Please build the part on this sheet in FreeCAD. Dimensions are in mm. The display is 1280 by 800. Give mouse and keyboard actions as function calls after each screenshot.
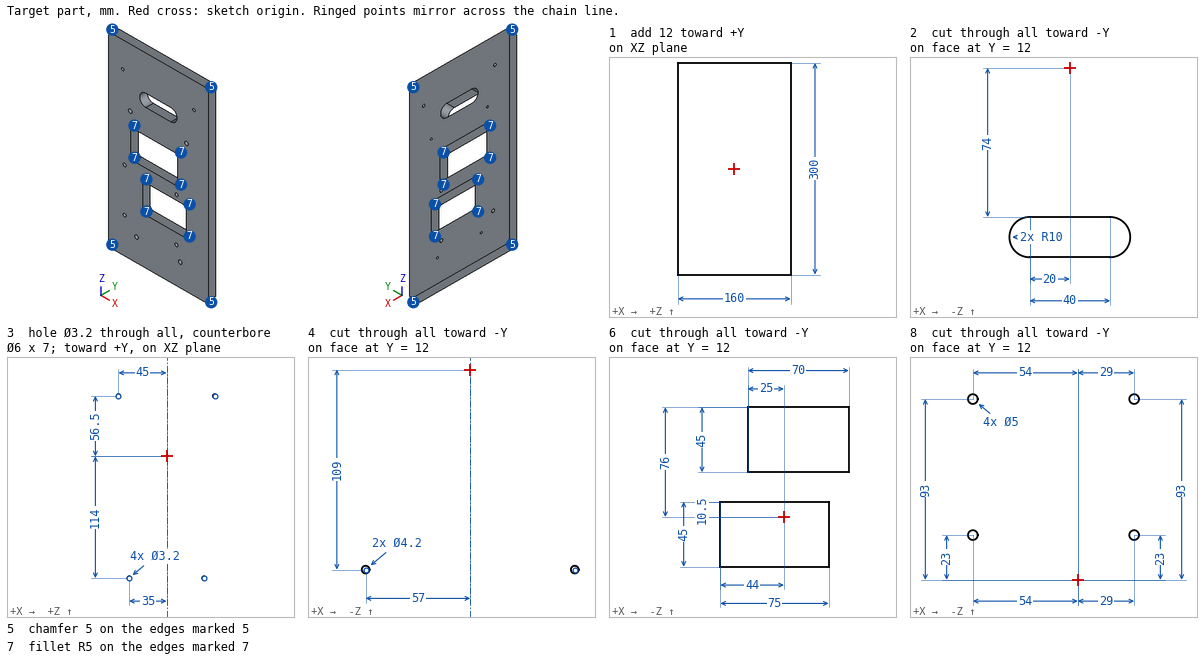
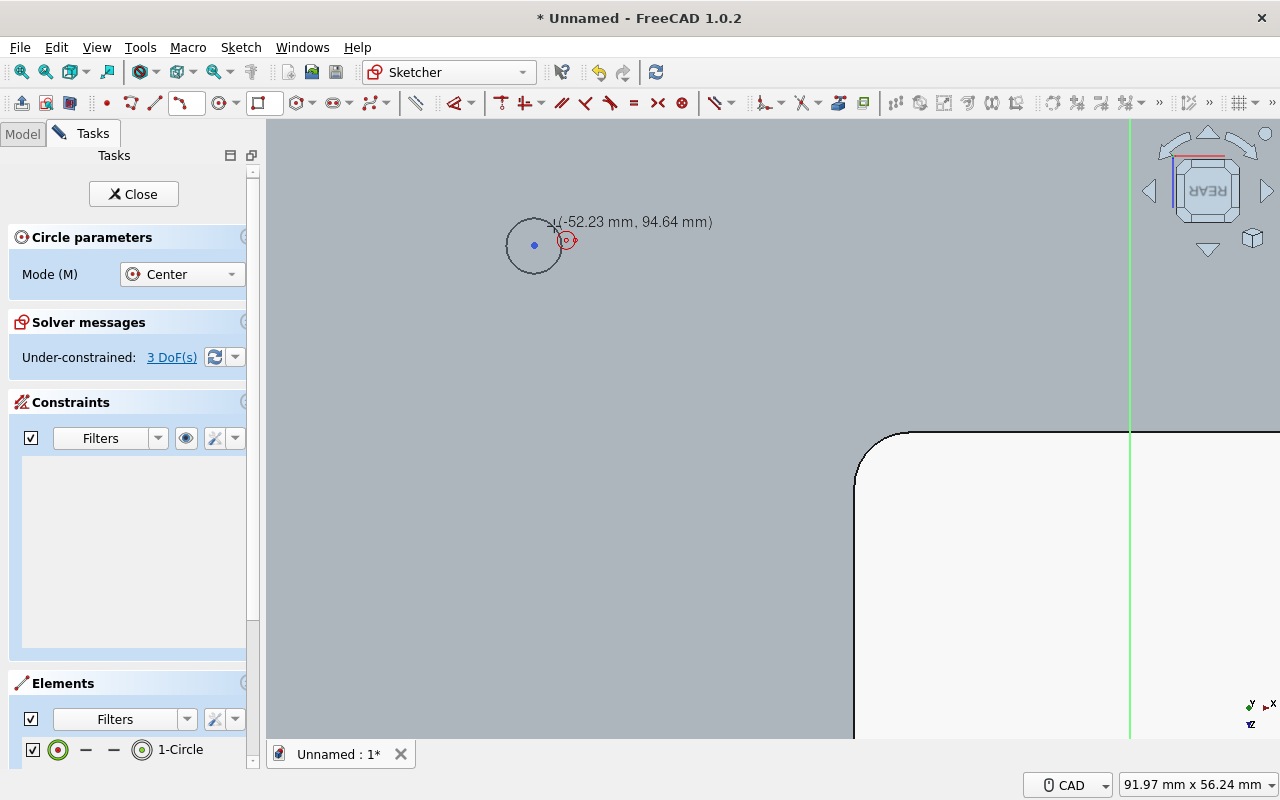
scroll(537, 246, down, 5)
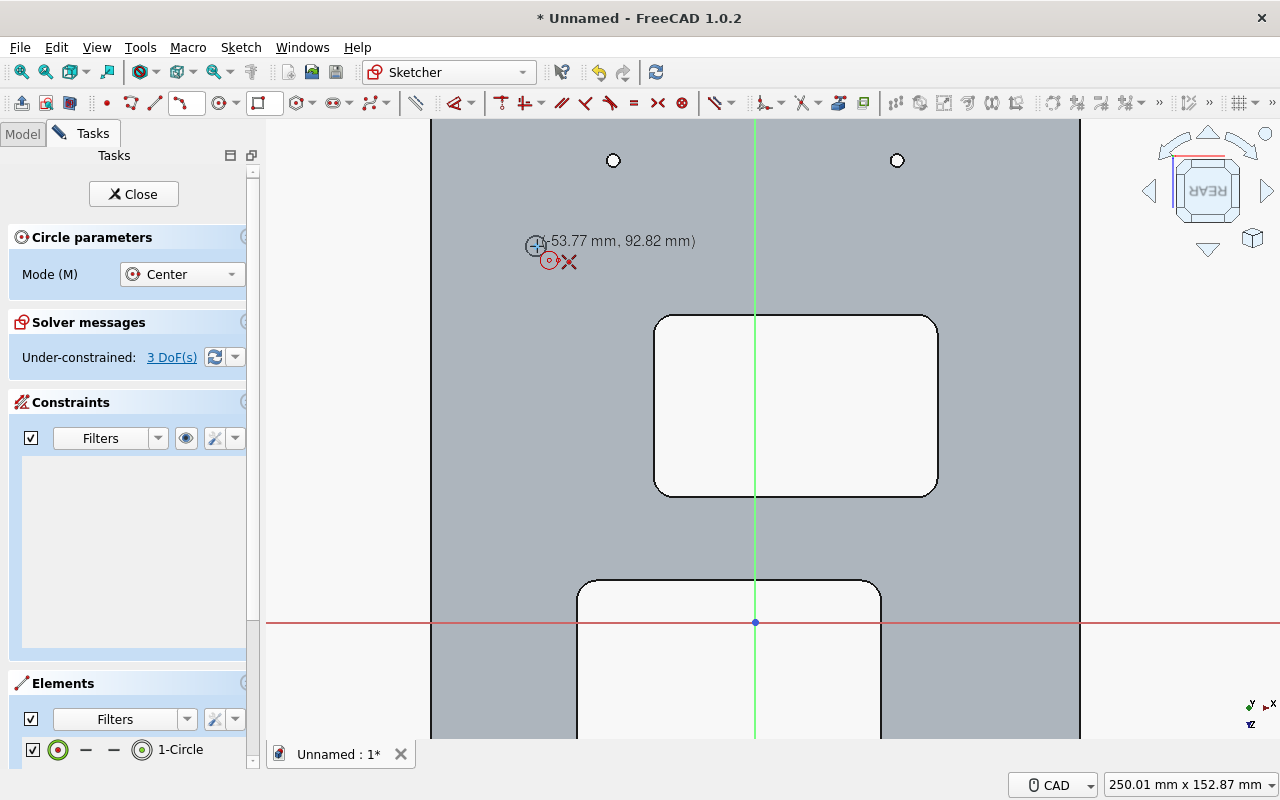
scroll(873, 246, up, 5)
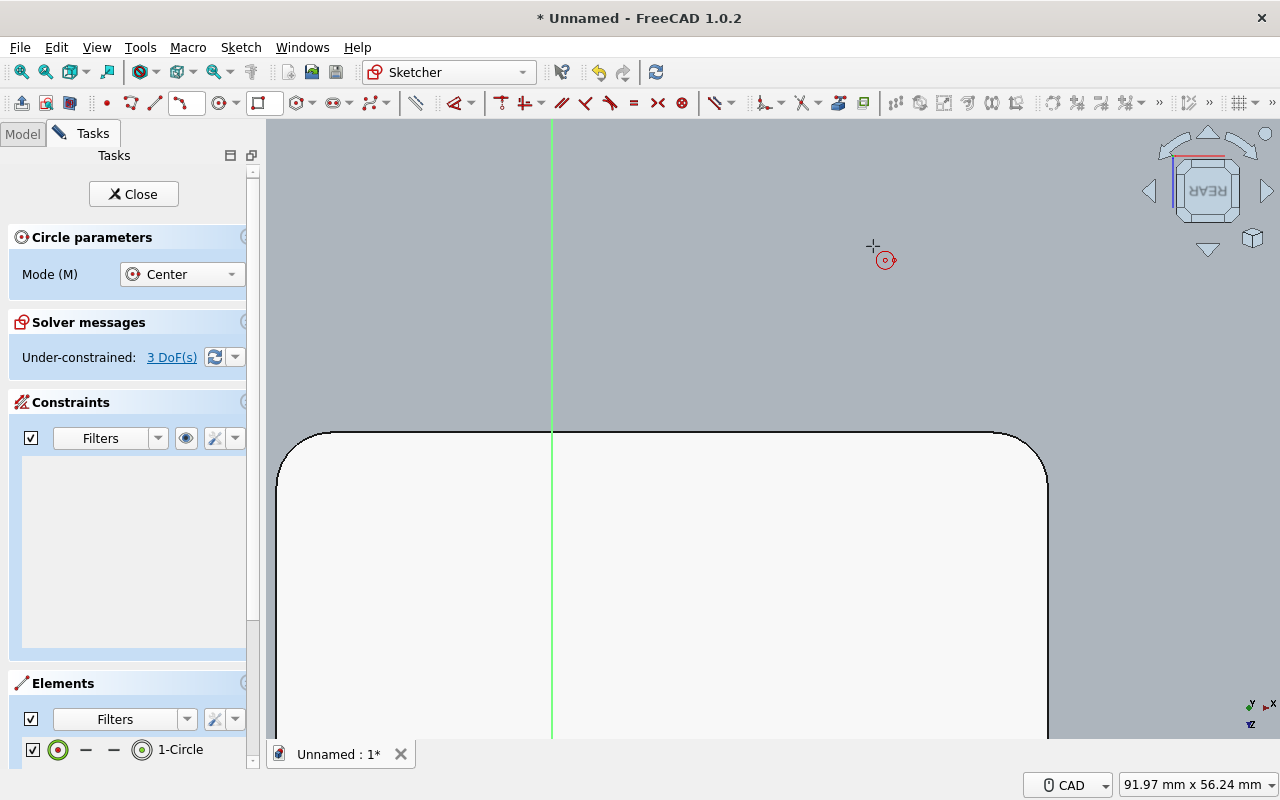
click(872, 245)
click(891, 226)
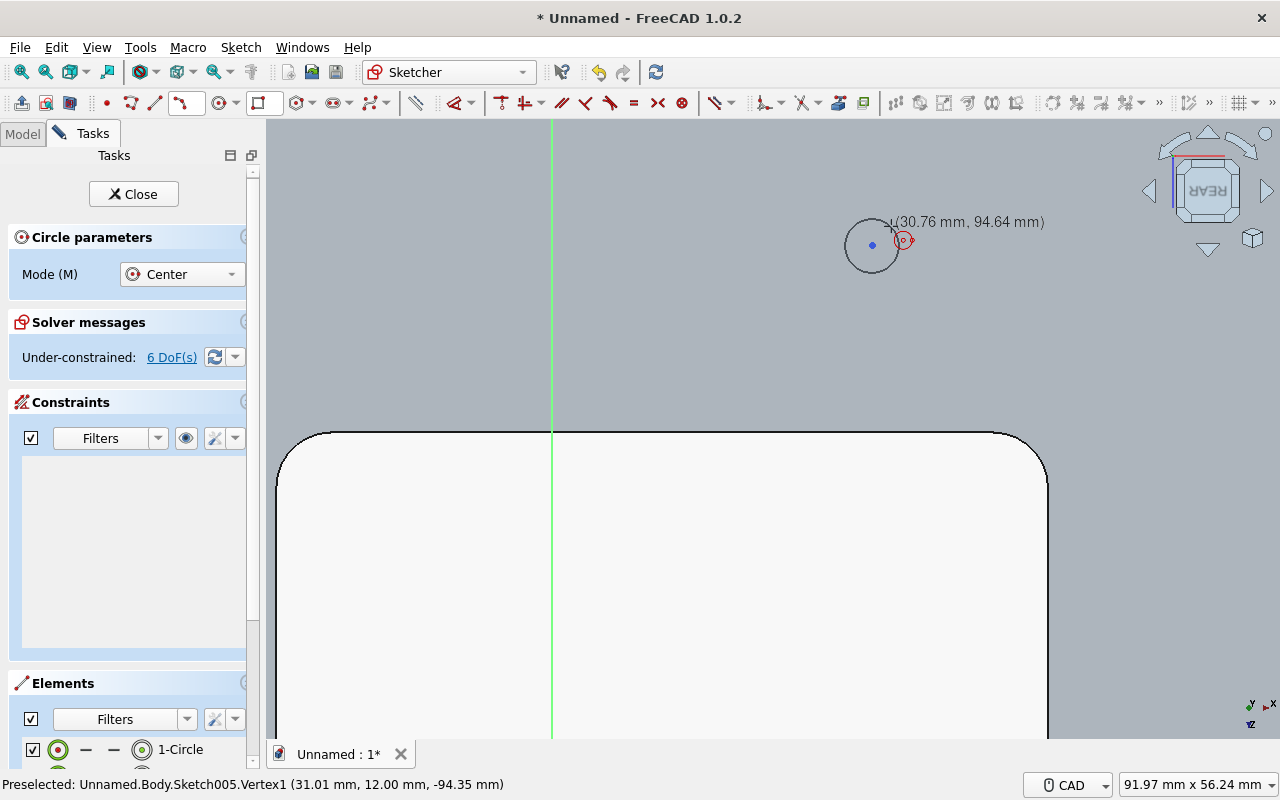
scroll(874, 246, down, 5)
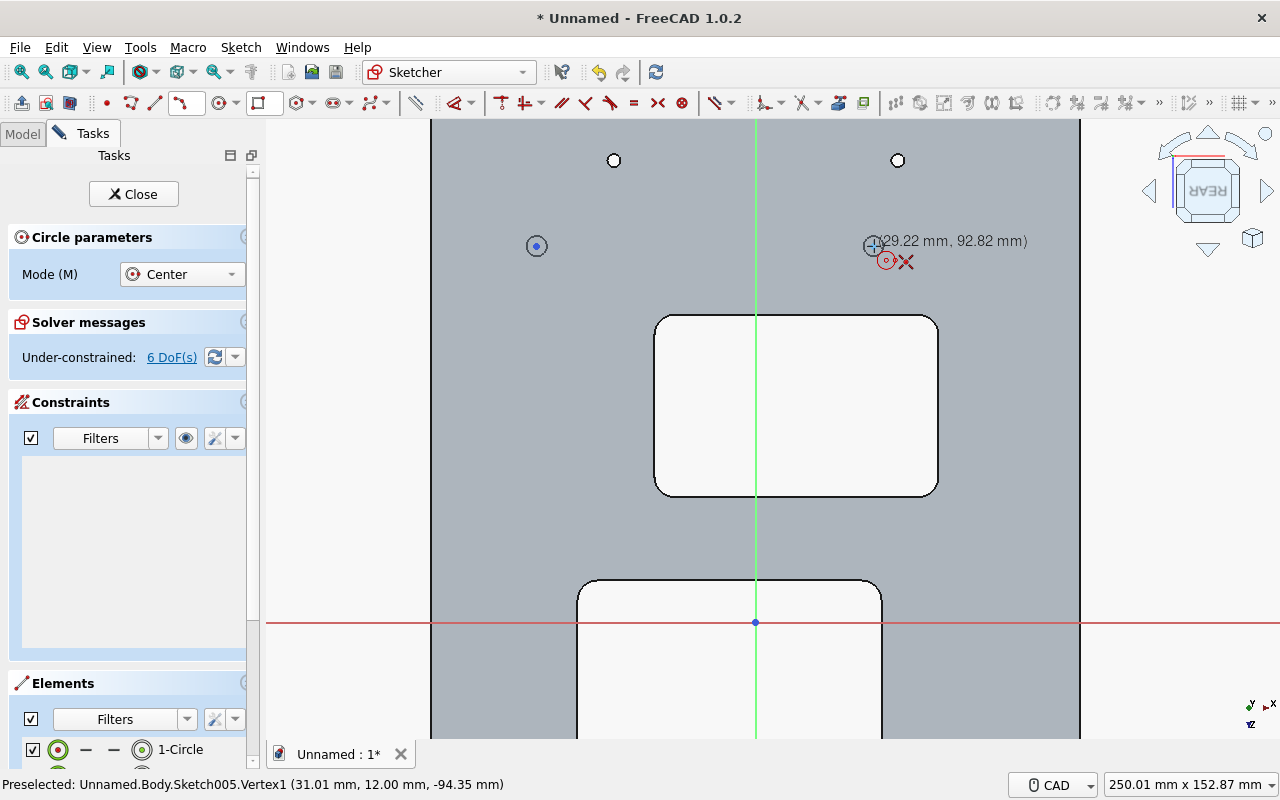
scroll(537, 530, up, 5)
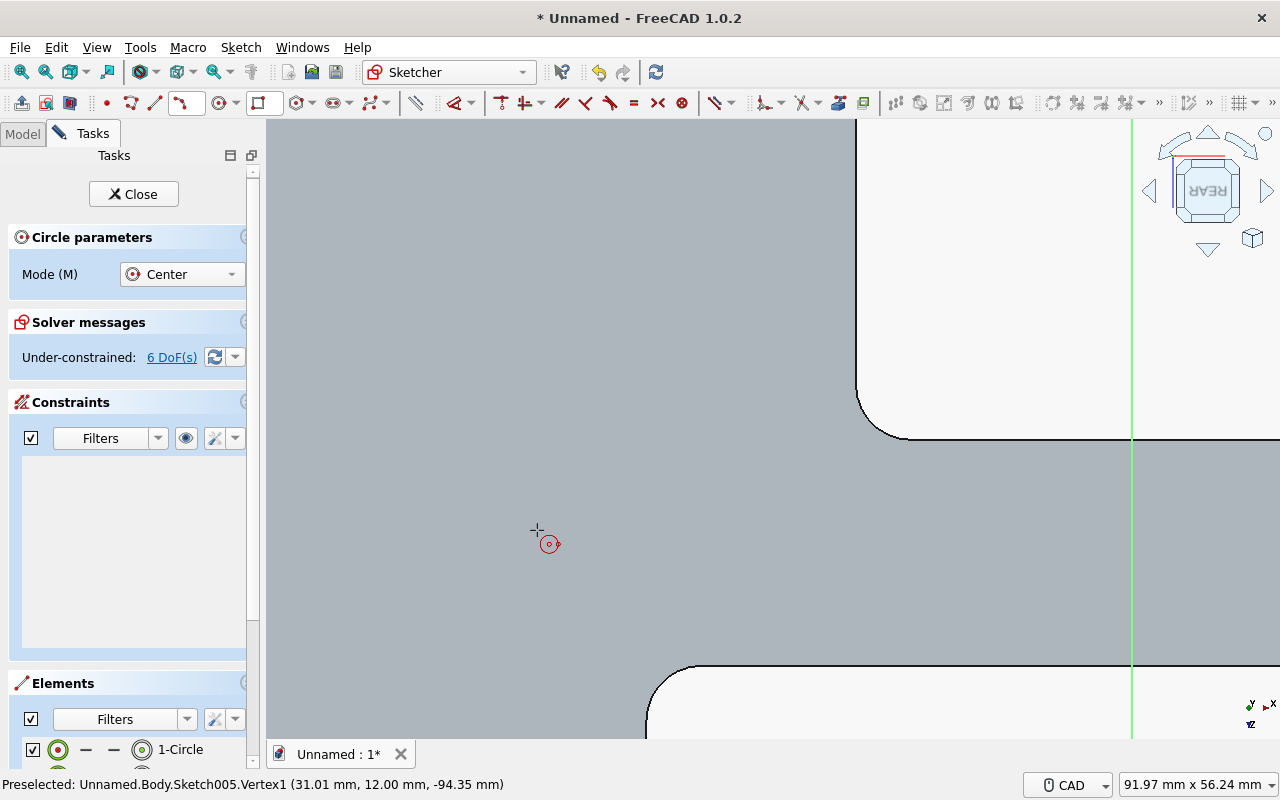
click(536, 528)
click(556, 509)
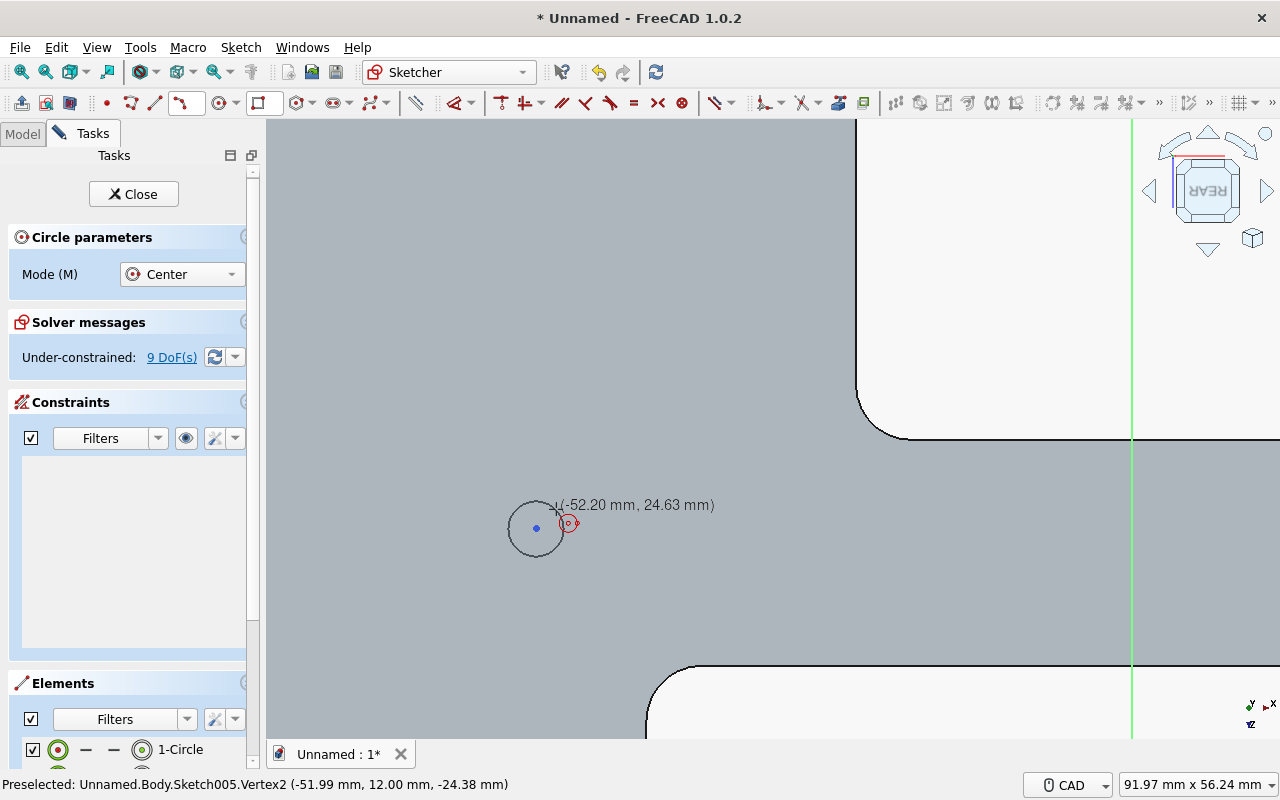
scroll(536, 530, down, 5)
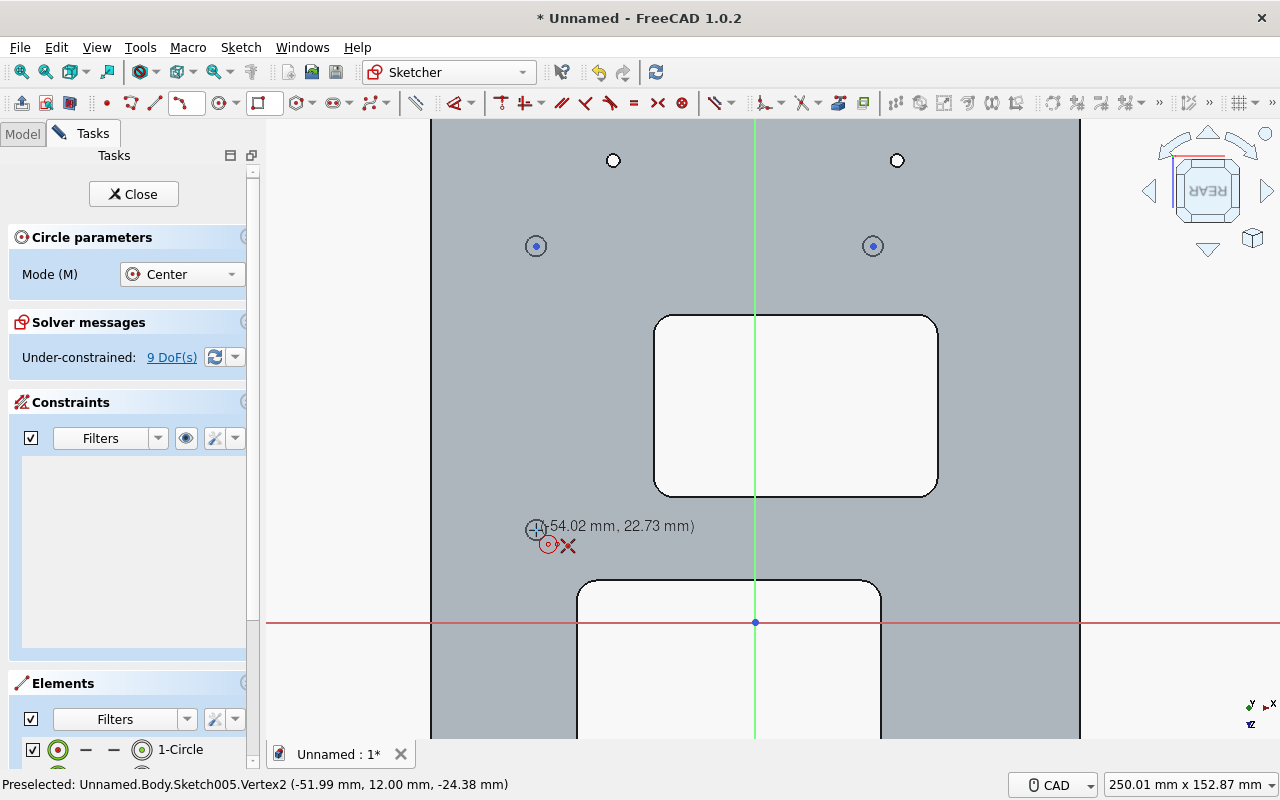
scroll(873, 530, up, 5)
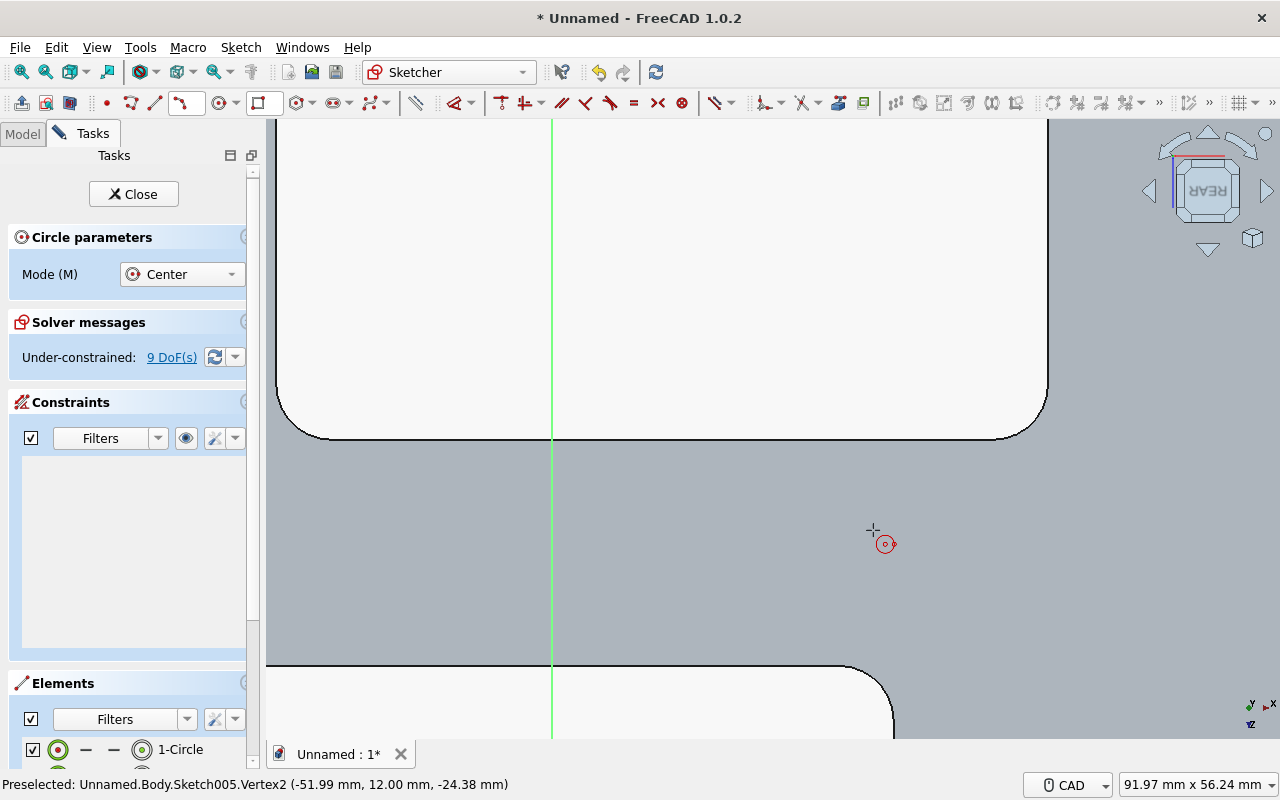
click(872, 528)
click(891, 509)
key(Escape)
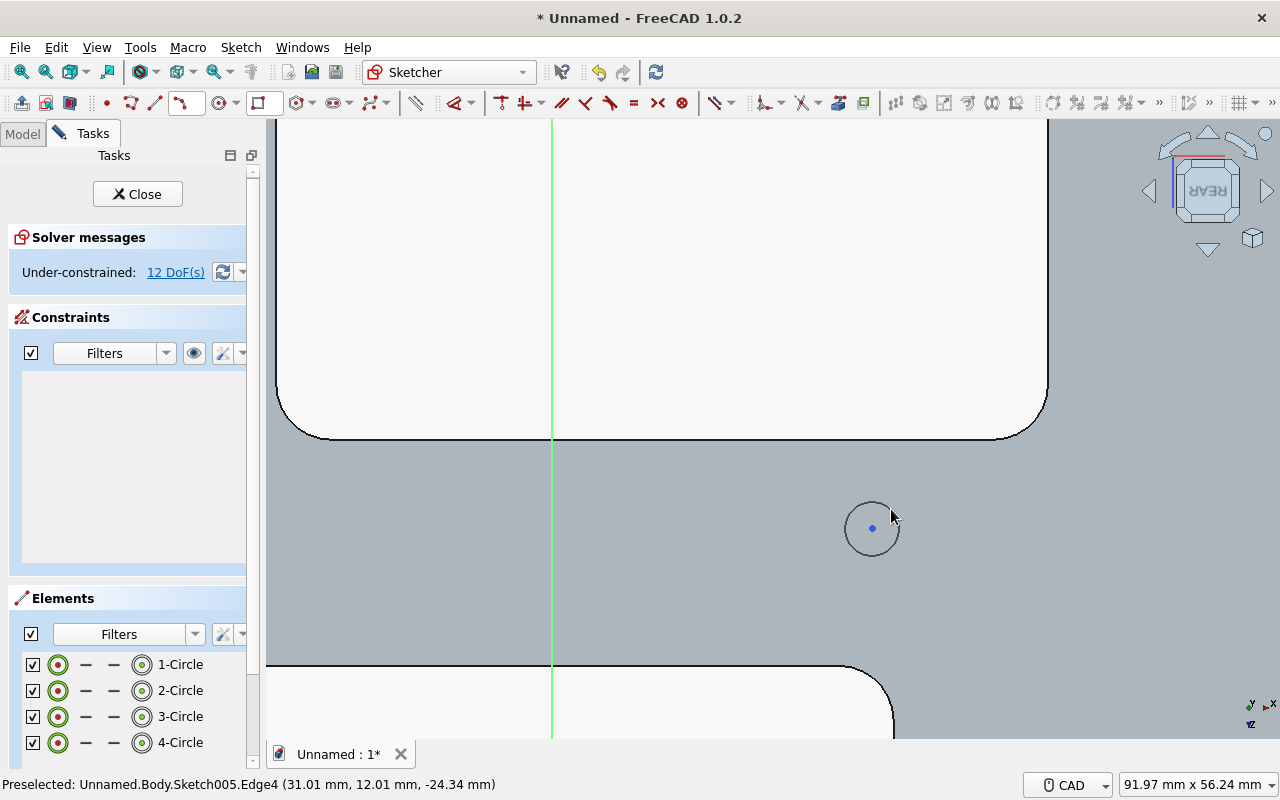
scroll(874, 530, down, 5)